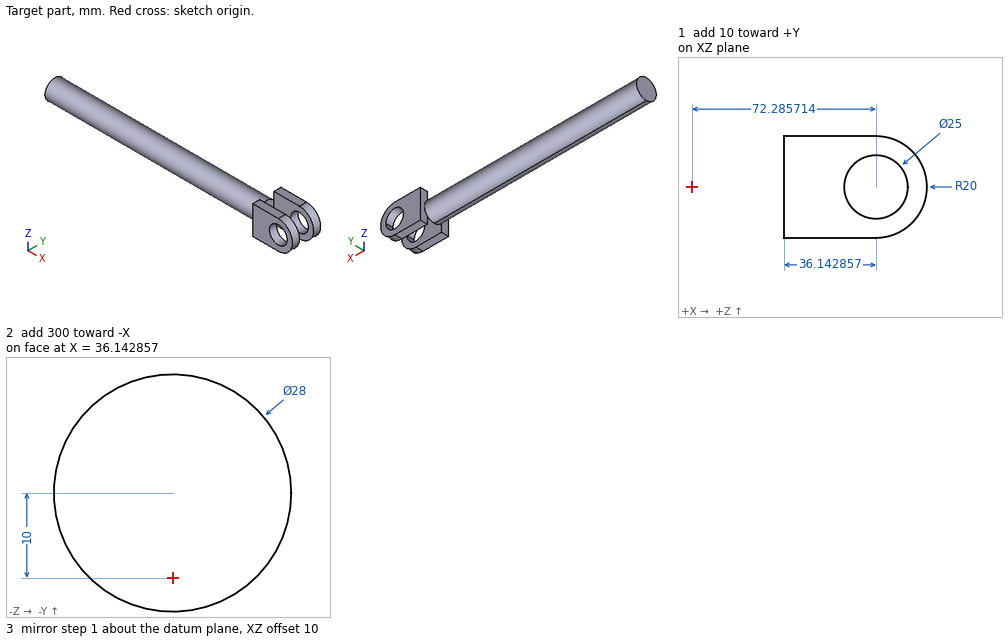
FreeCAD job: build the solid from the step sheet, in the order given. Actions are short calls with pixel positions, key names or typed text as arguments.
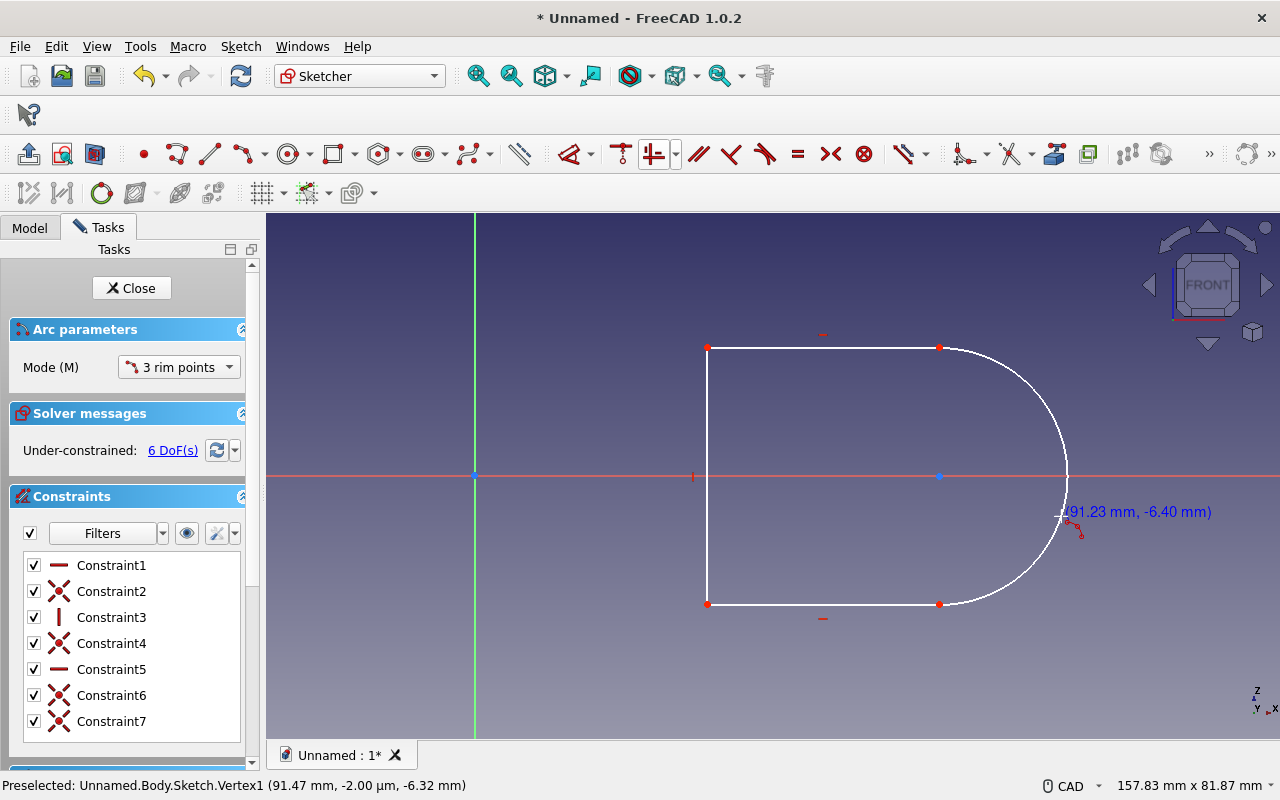
key(g)
key(c)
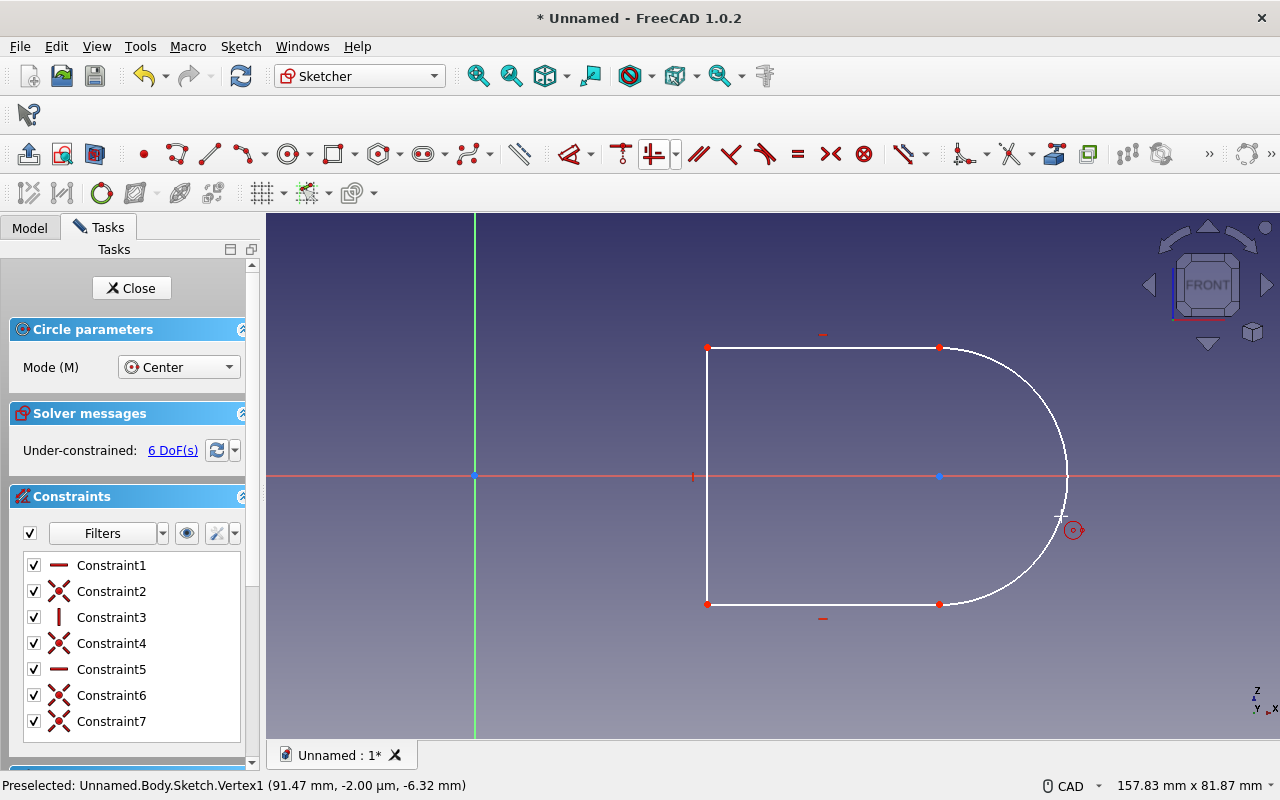
click(939, 476)
move(996, 419)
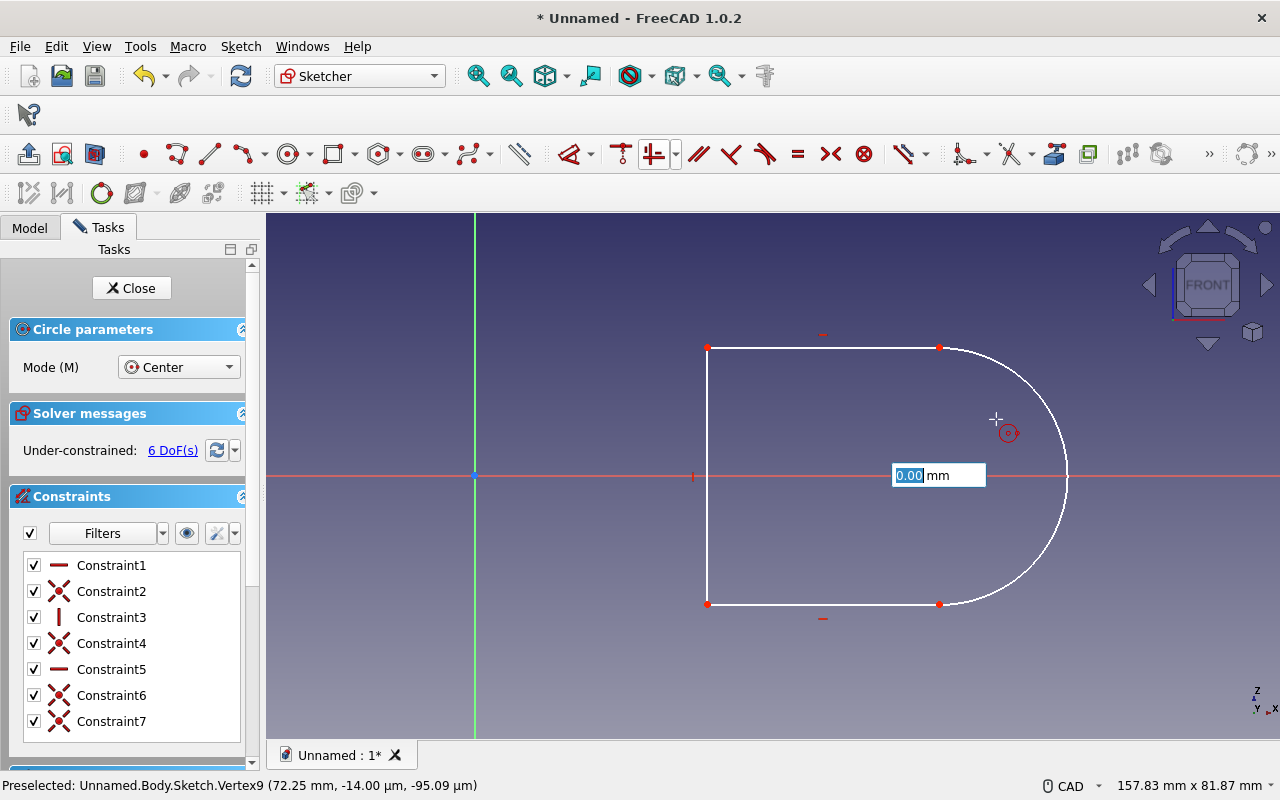
text(25)
key(Return)
key(Escape)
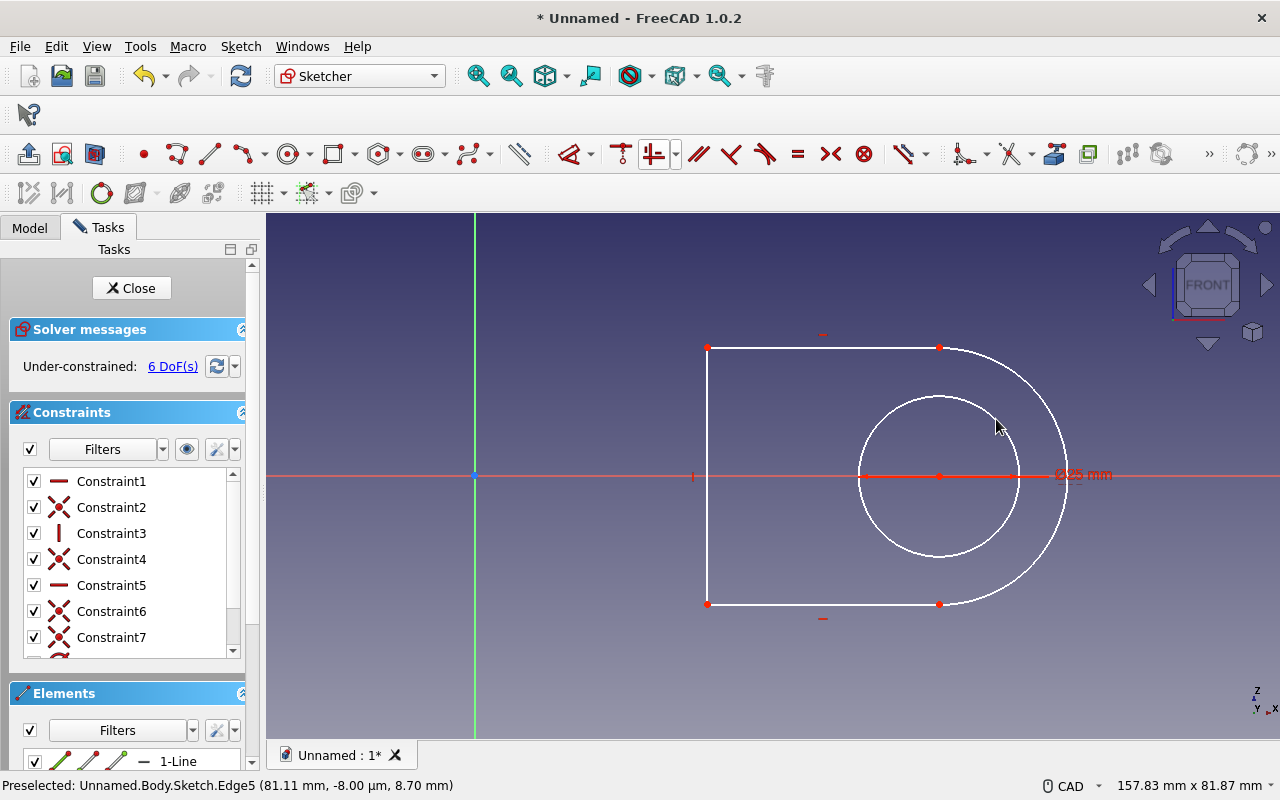
click(869, 605)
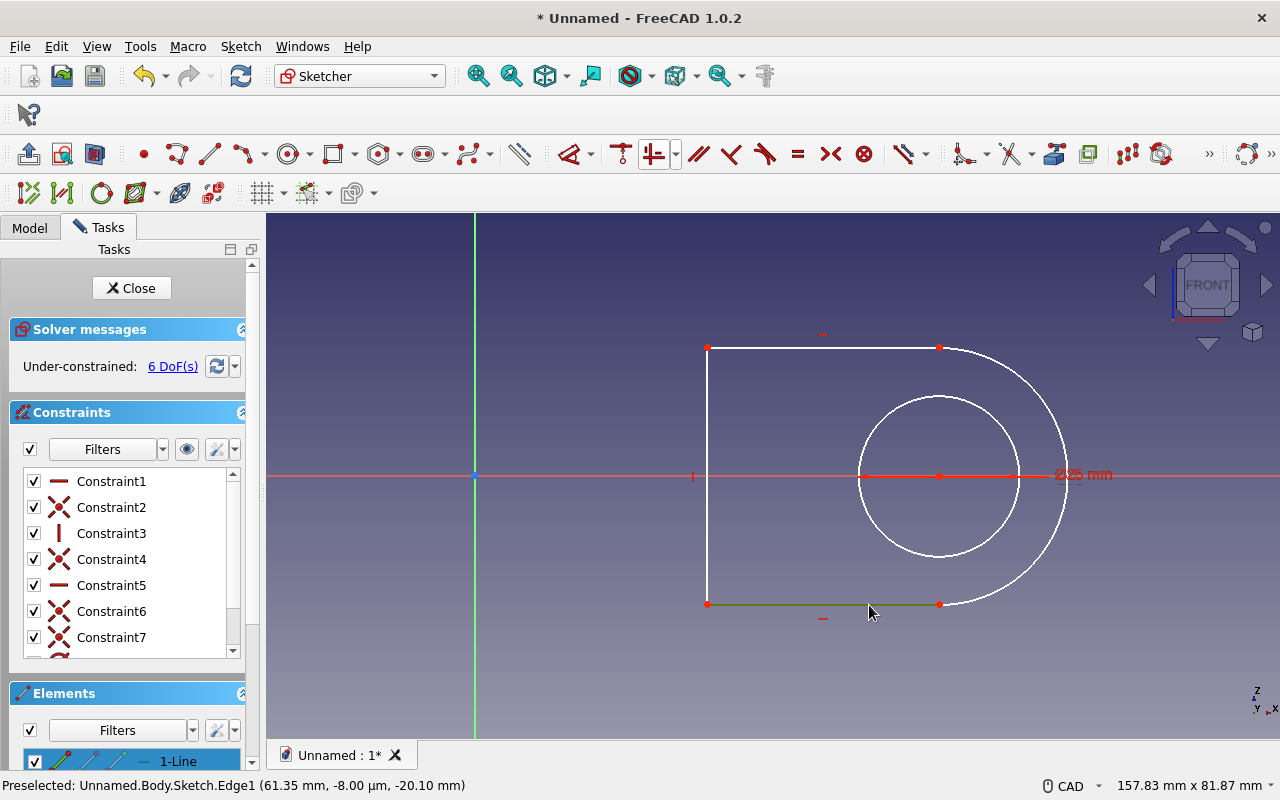
click(1043, 552)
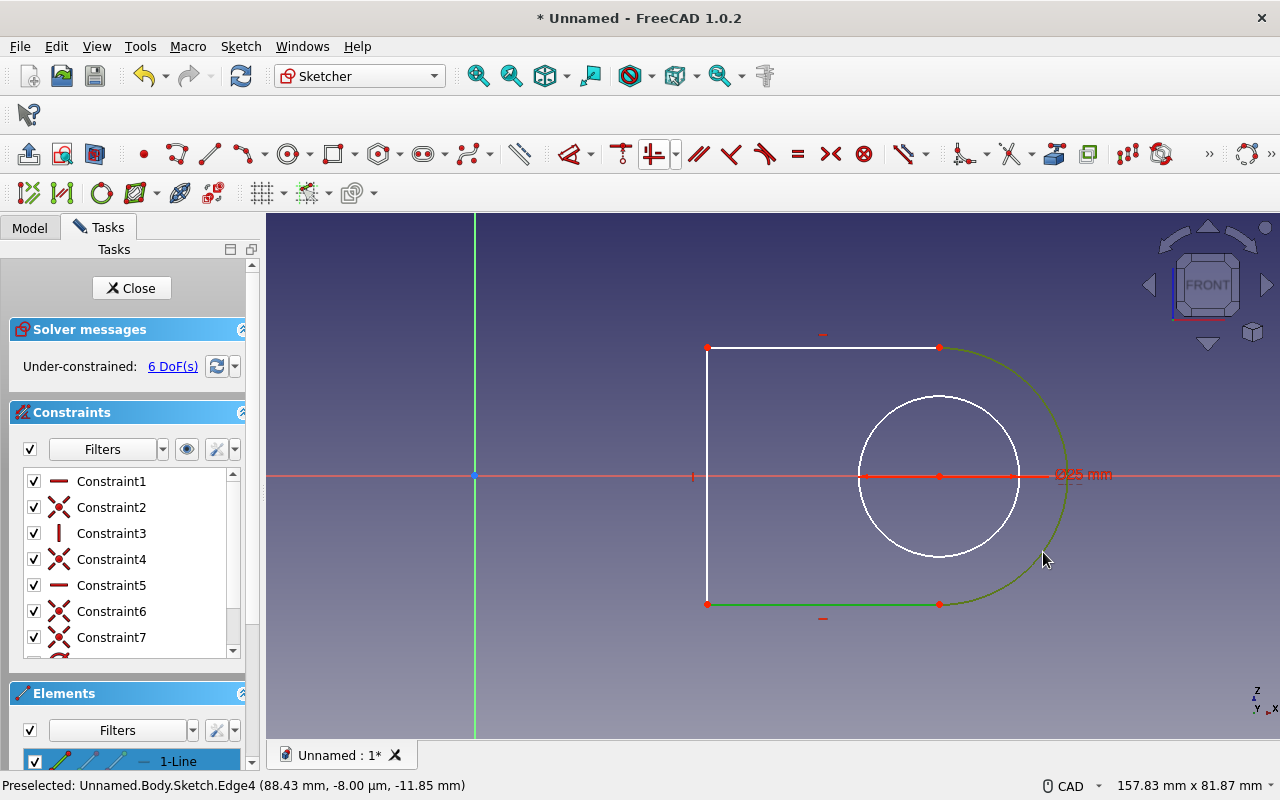
key(t)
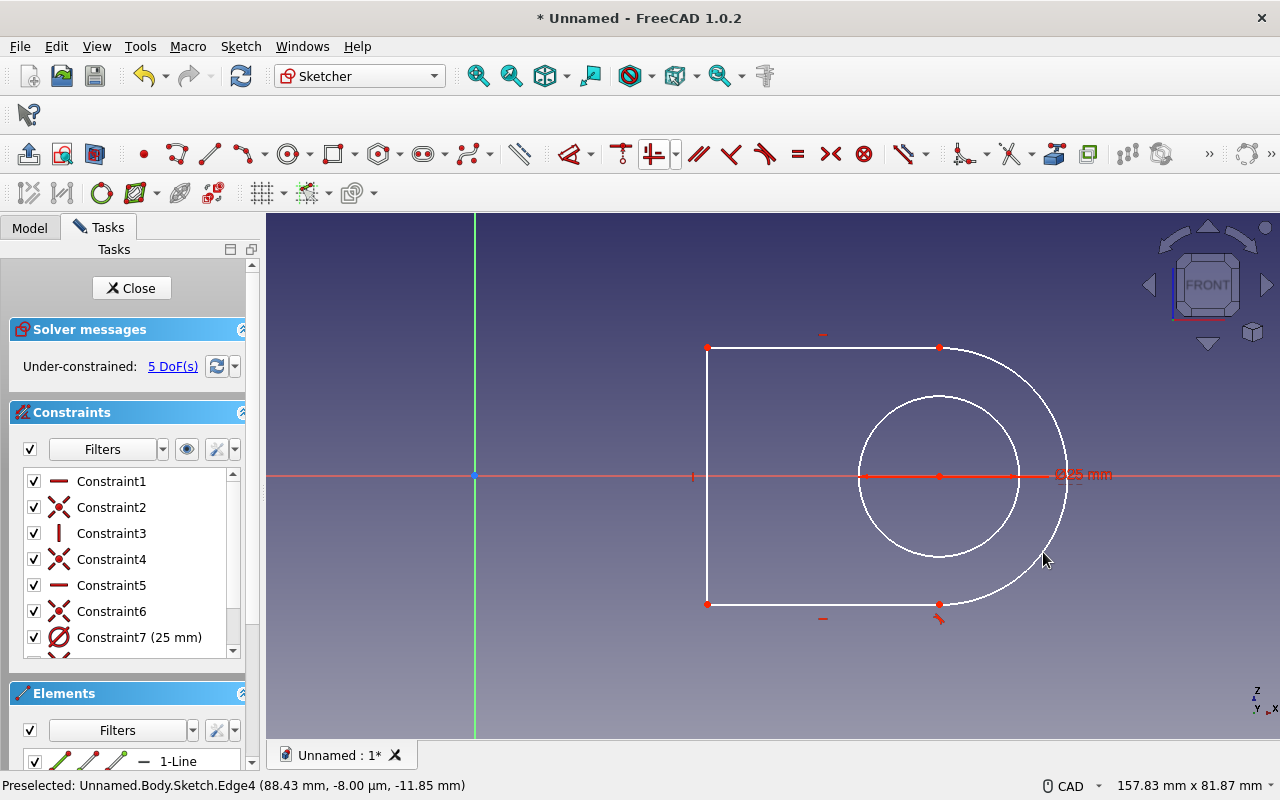
click(777, 348)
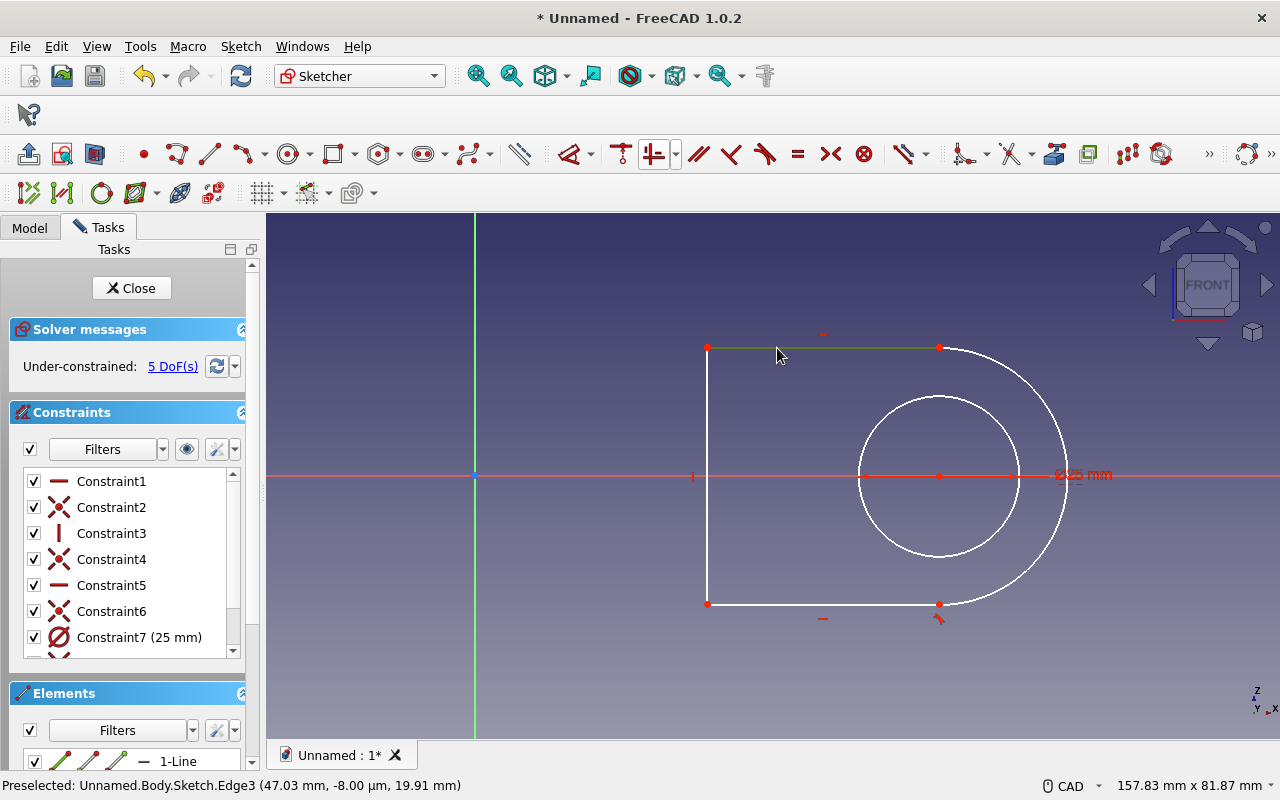
click(1043, 552)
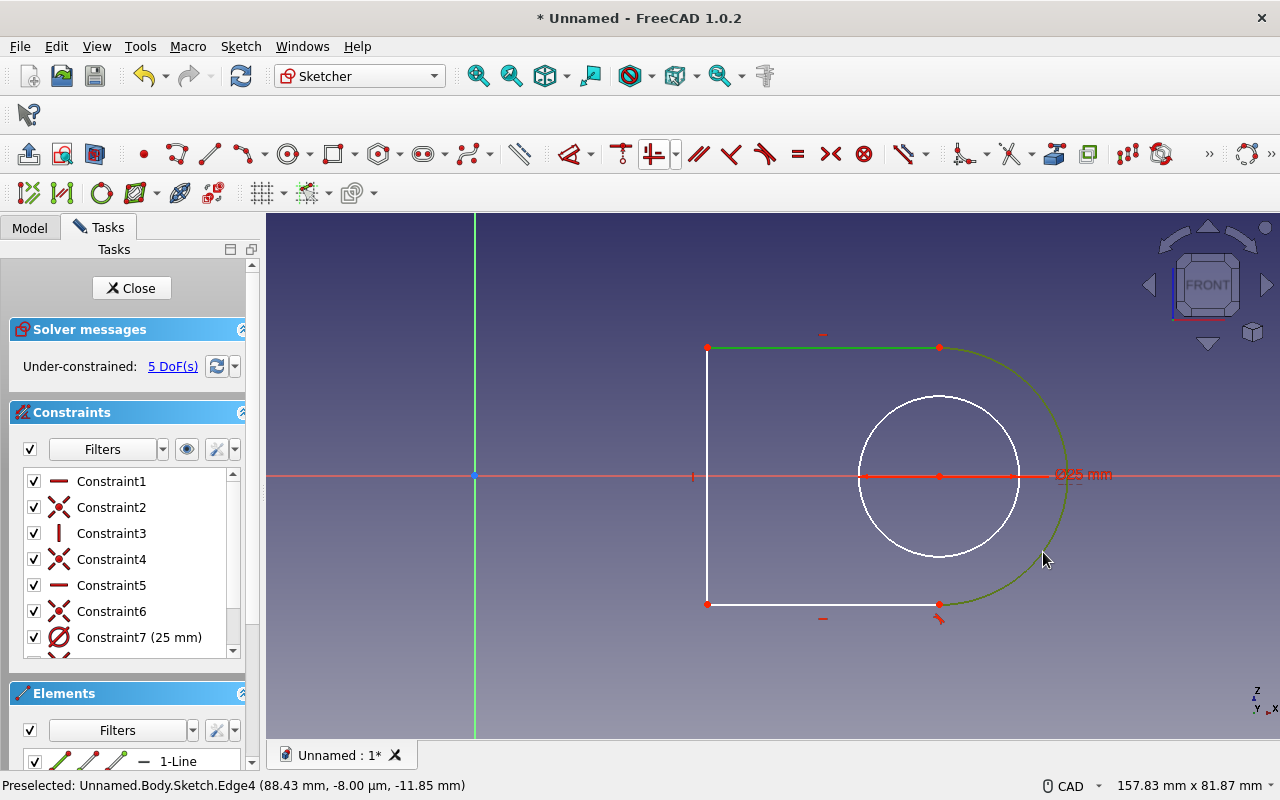
key(t)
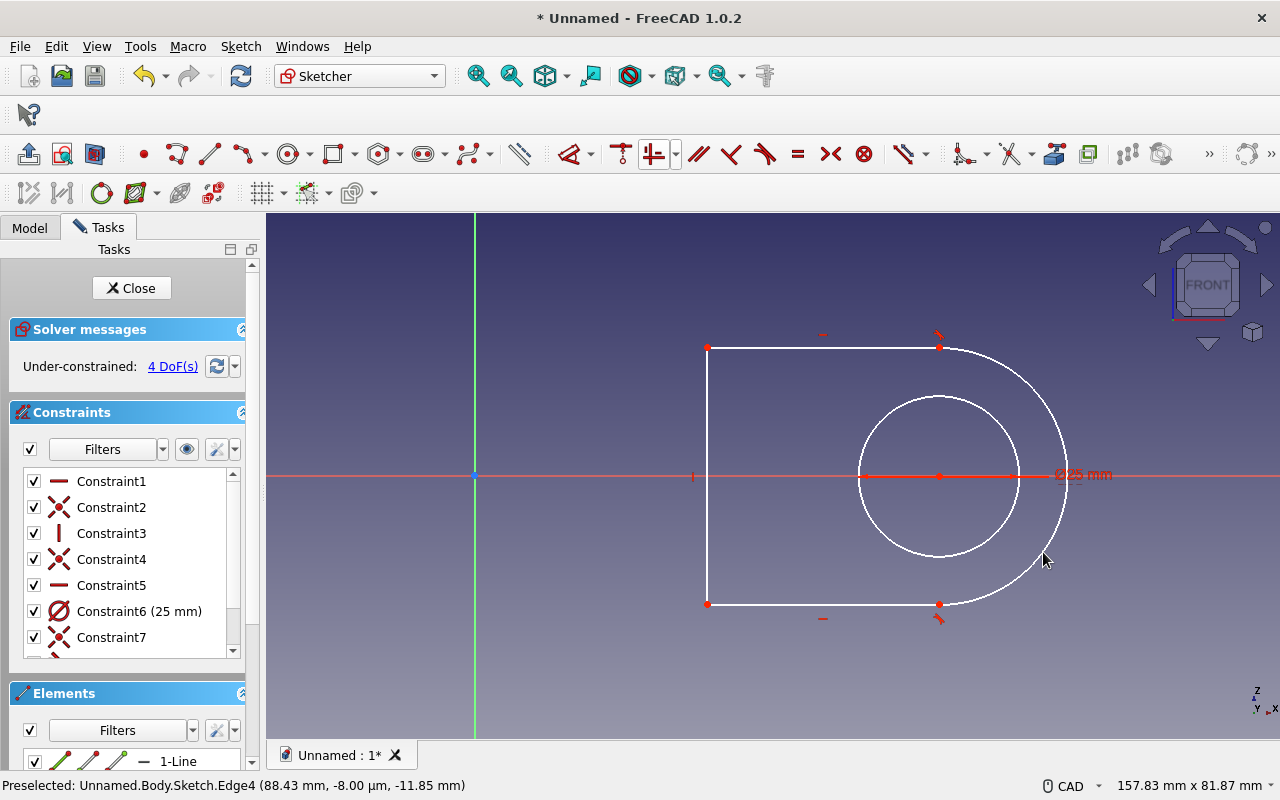
click(939, 476)